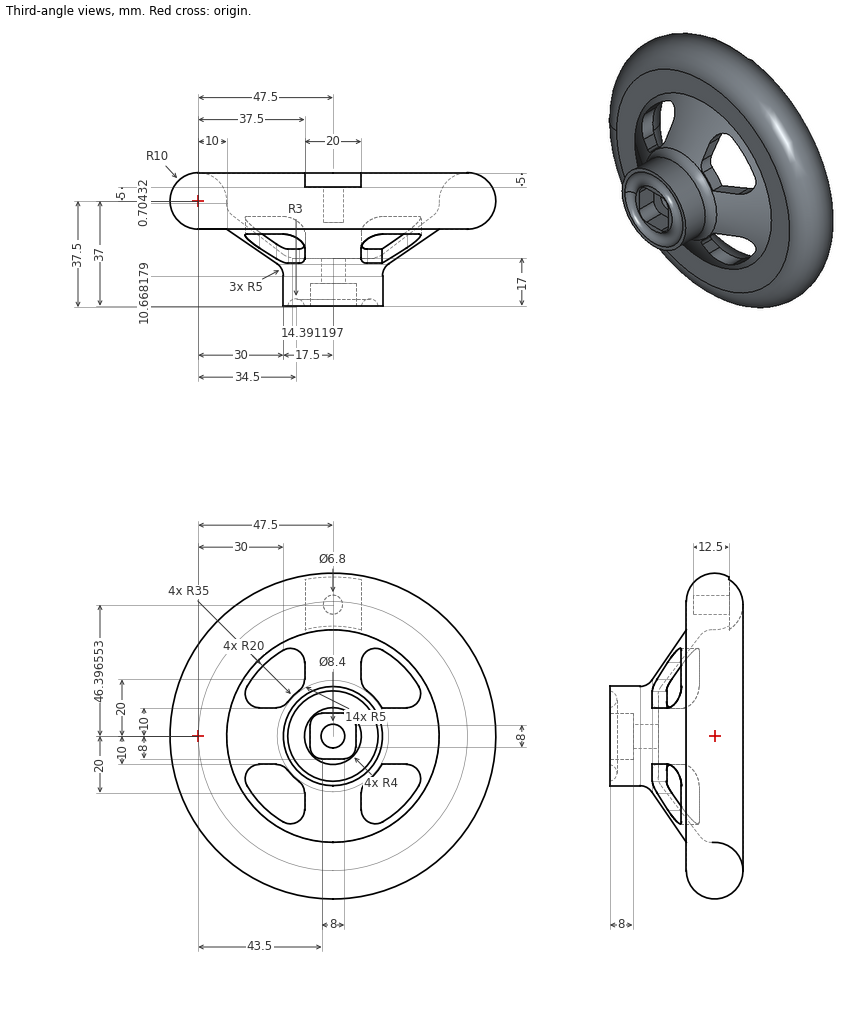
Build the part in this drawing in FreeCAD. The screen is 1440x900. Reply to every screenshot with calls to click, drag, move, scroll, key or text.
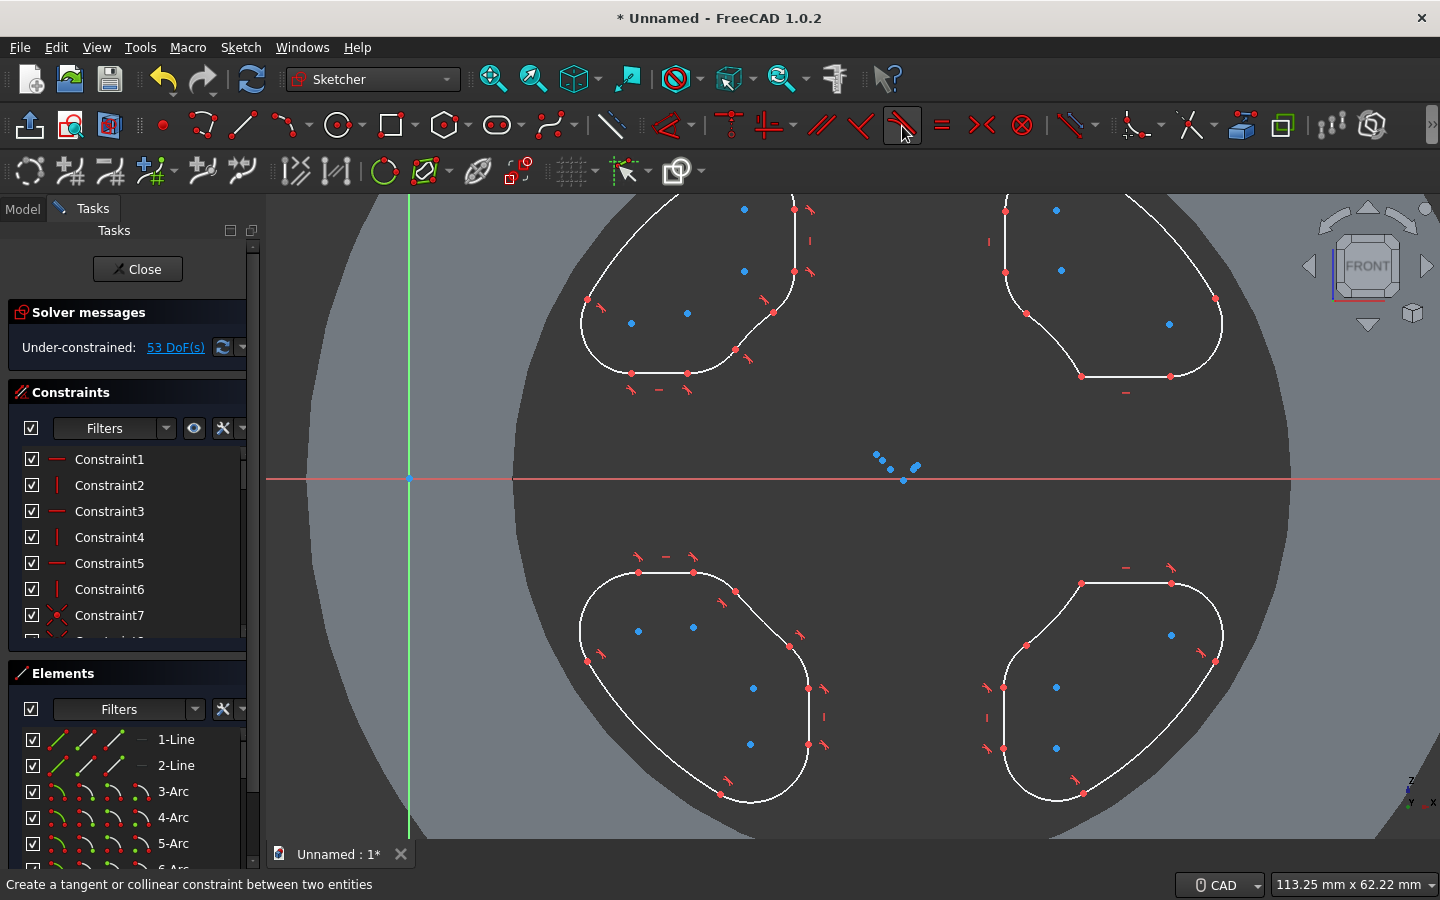
click(1015, 655)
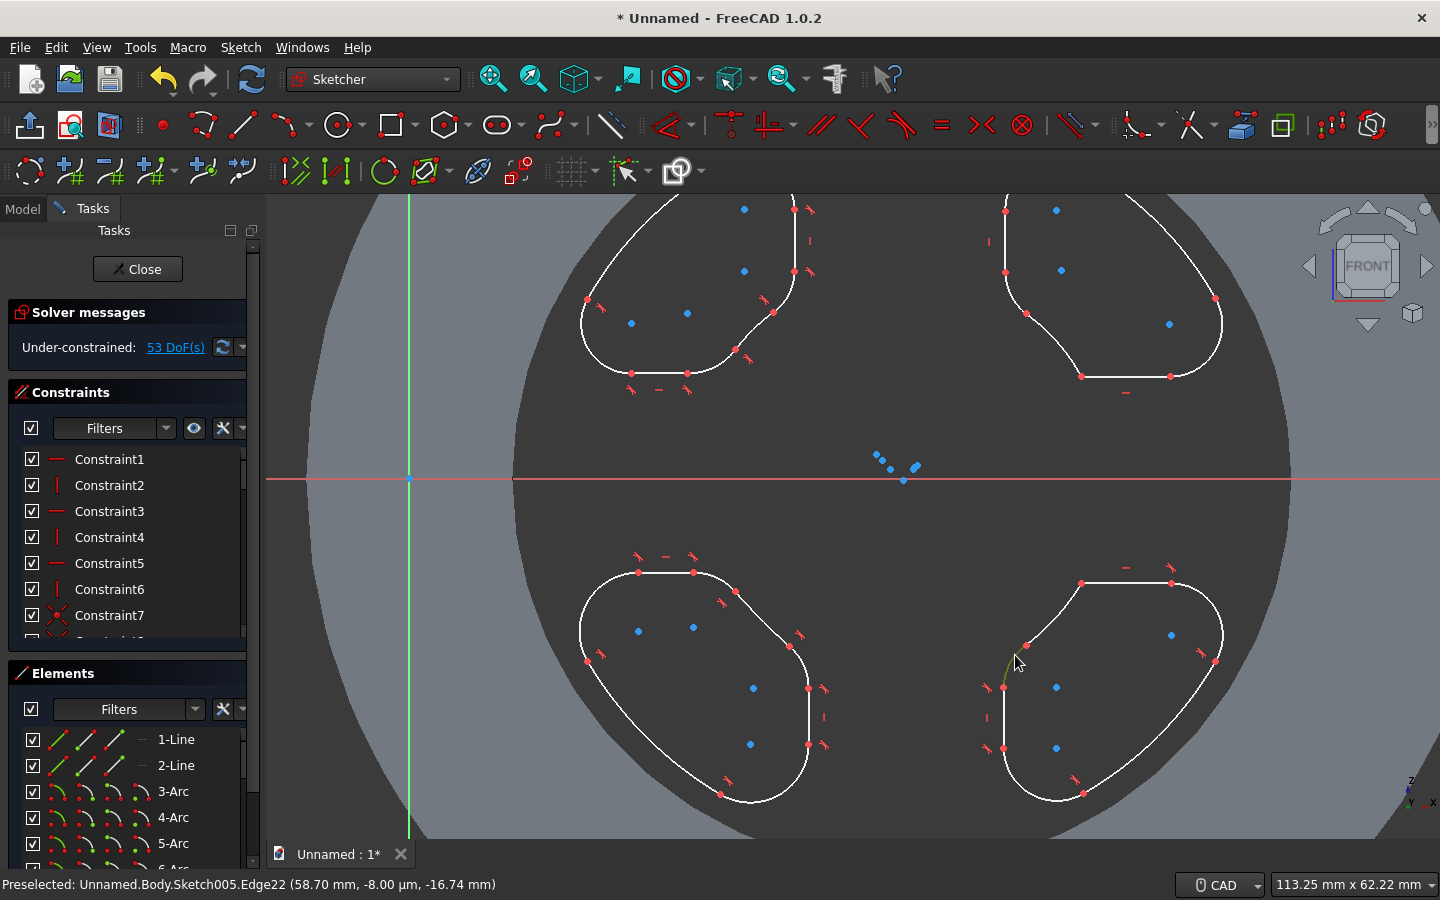
click(1045, 629)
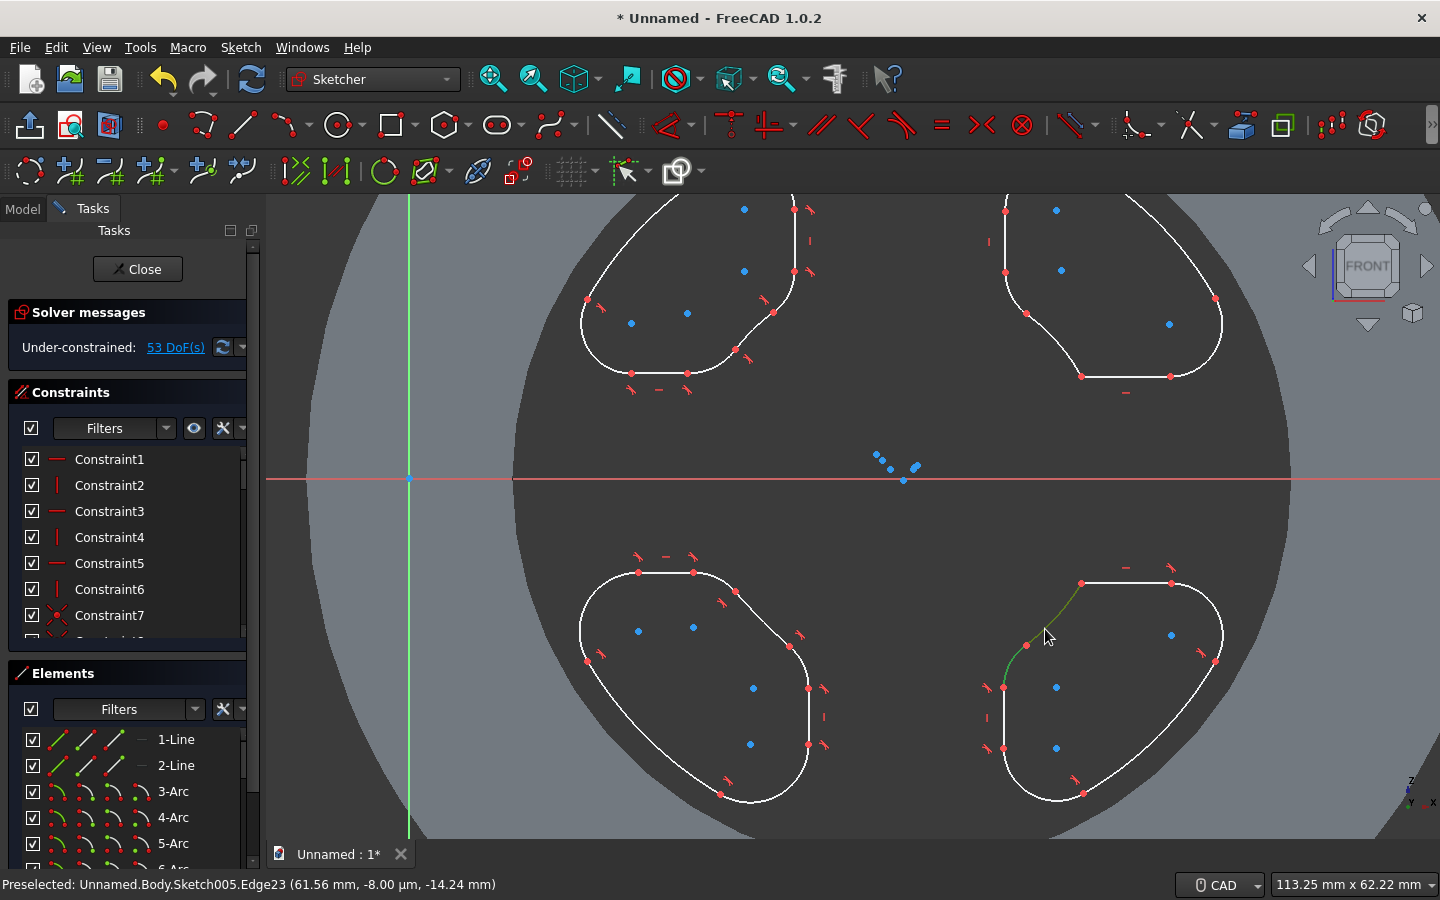
click(902, 126)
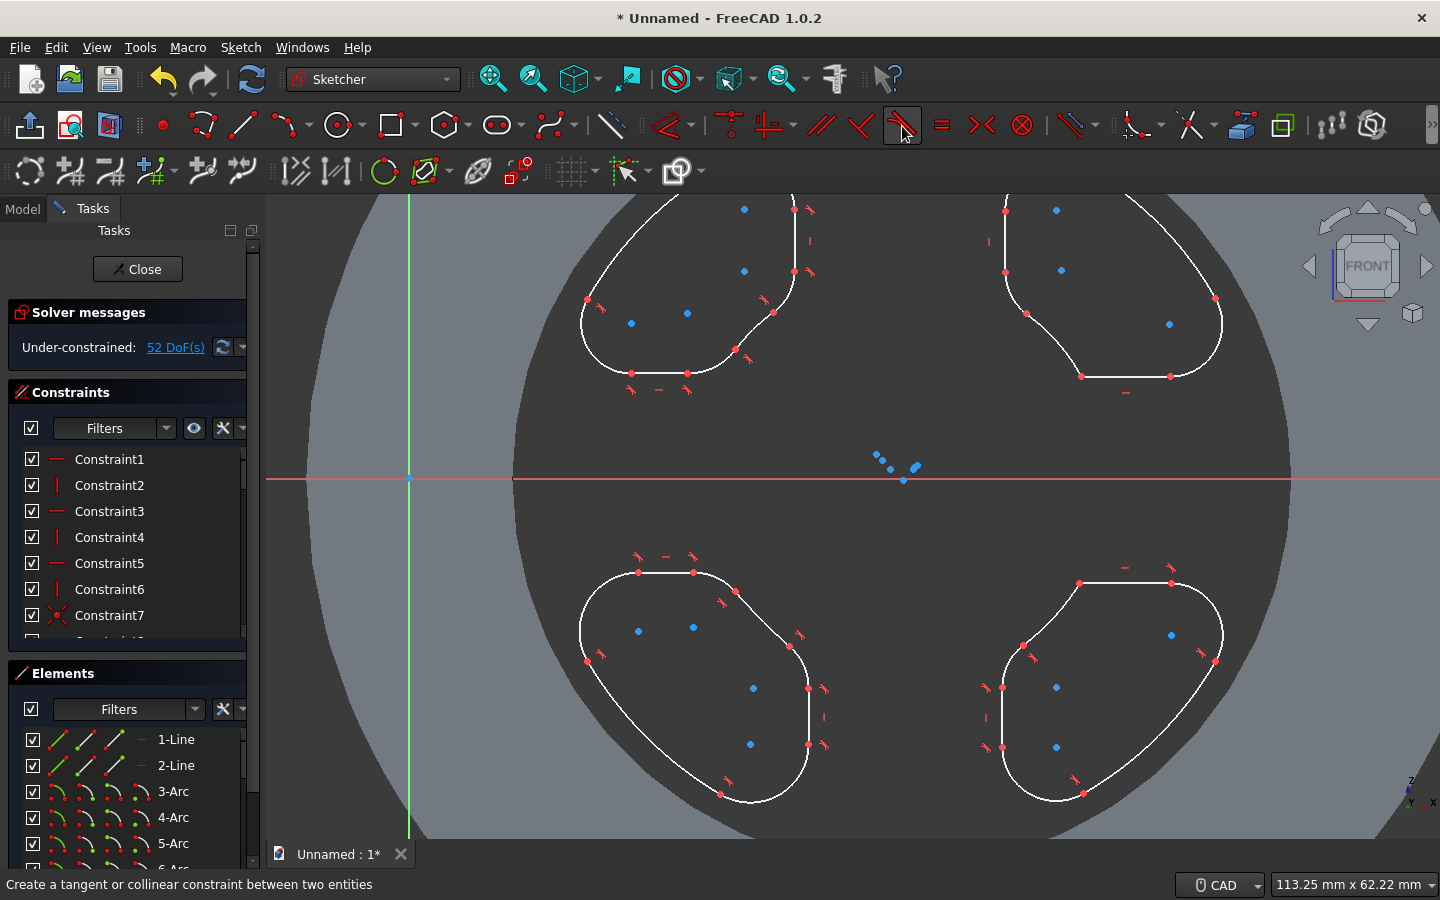
click(1144, 377)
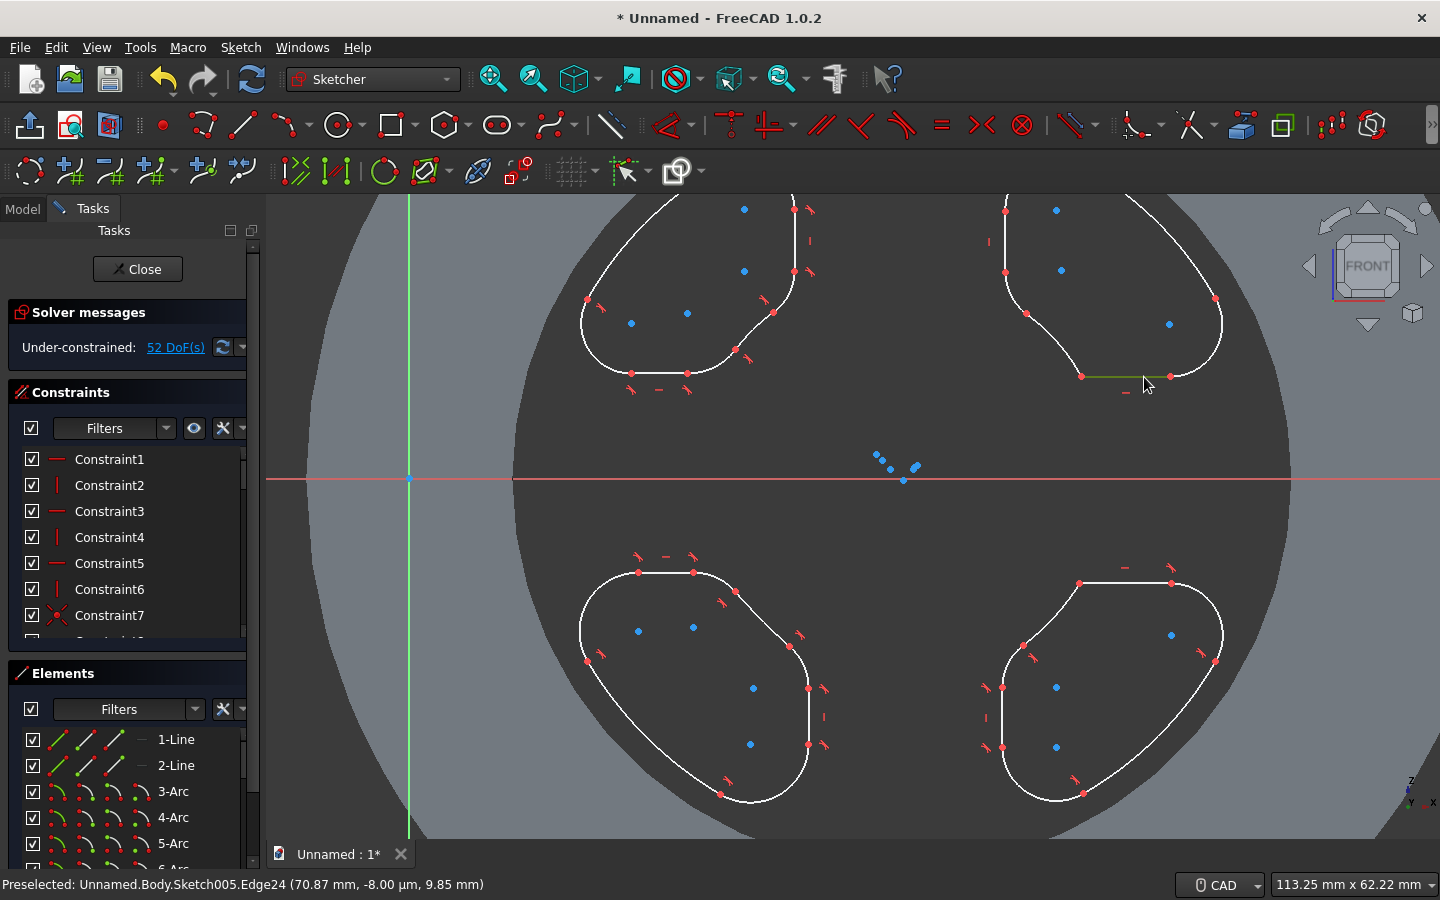
click(1201, 366)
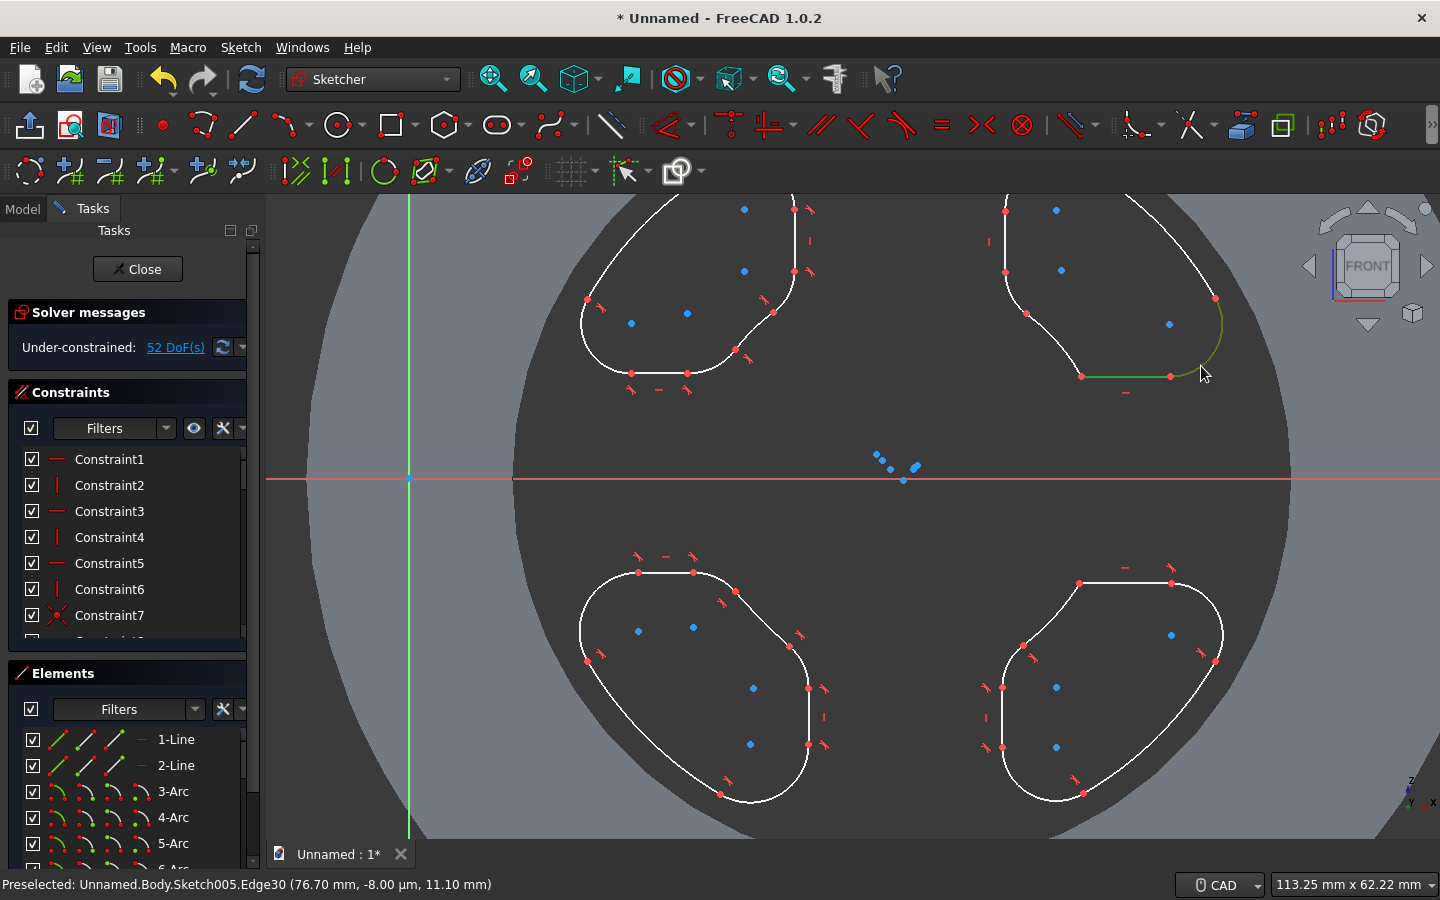
click(902, 126)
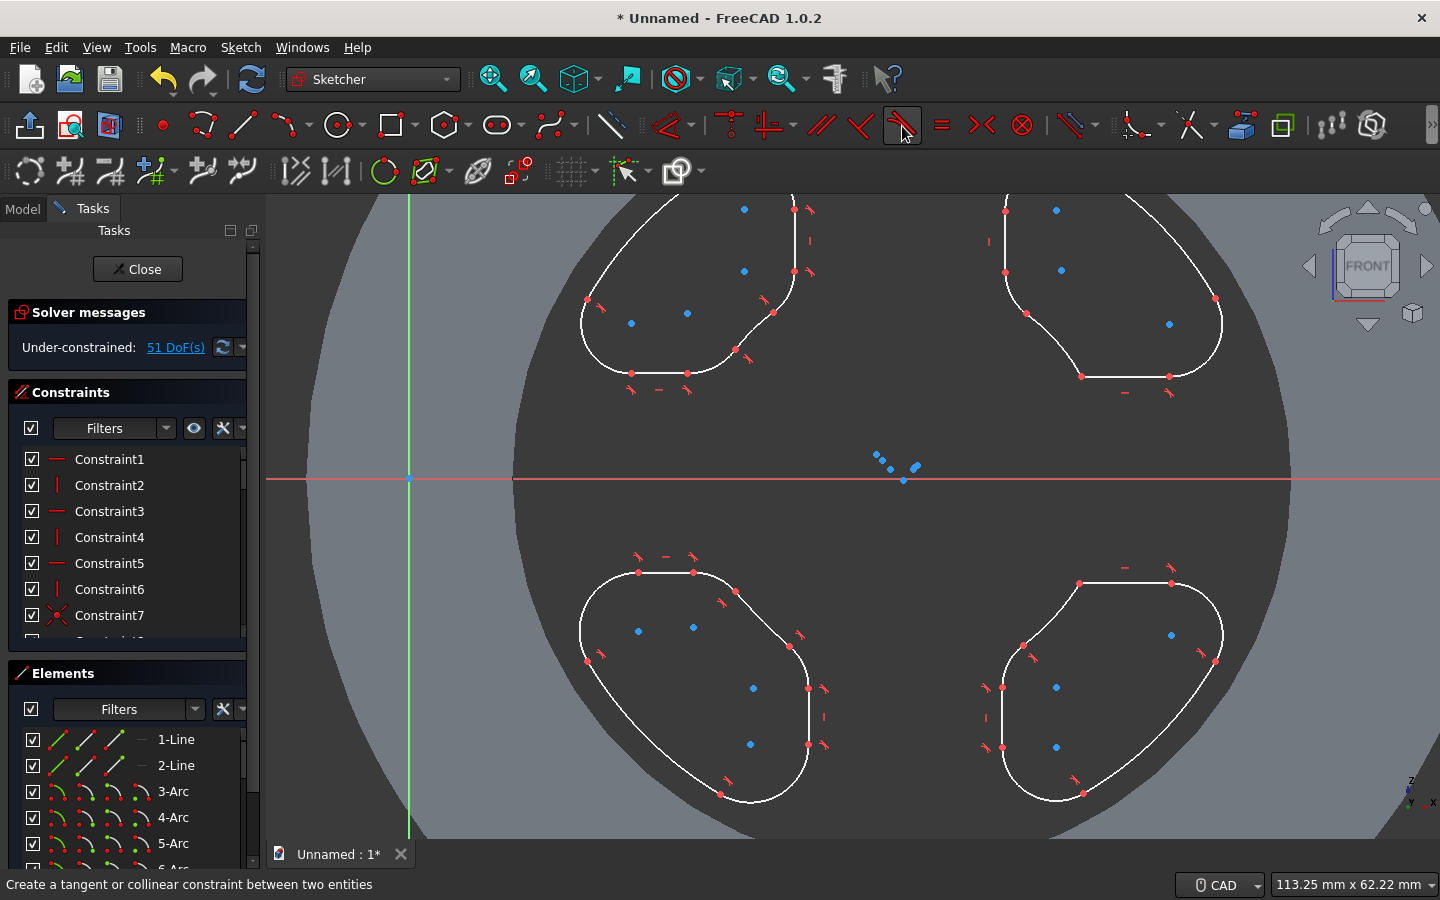
click(1005, 254)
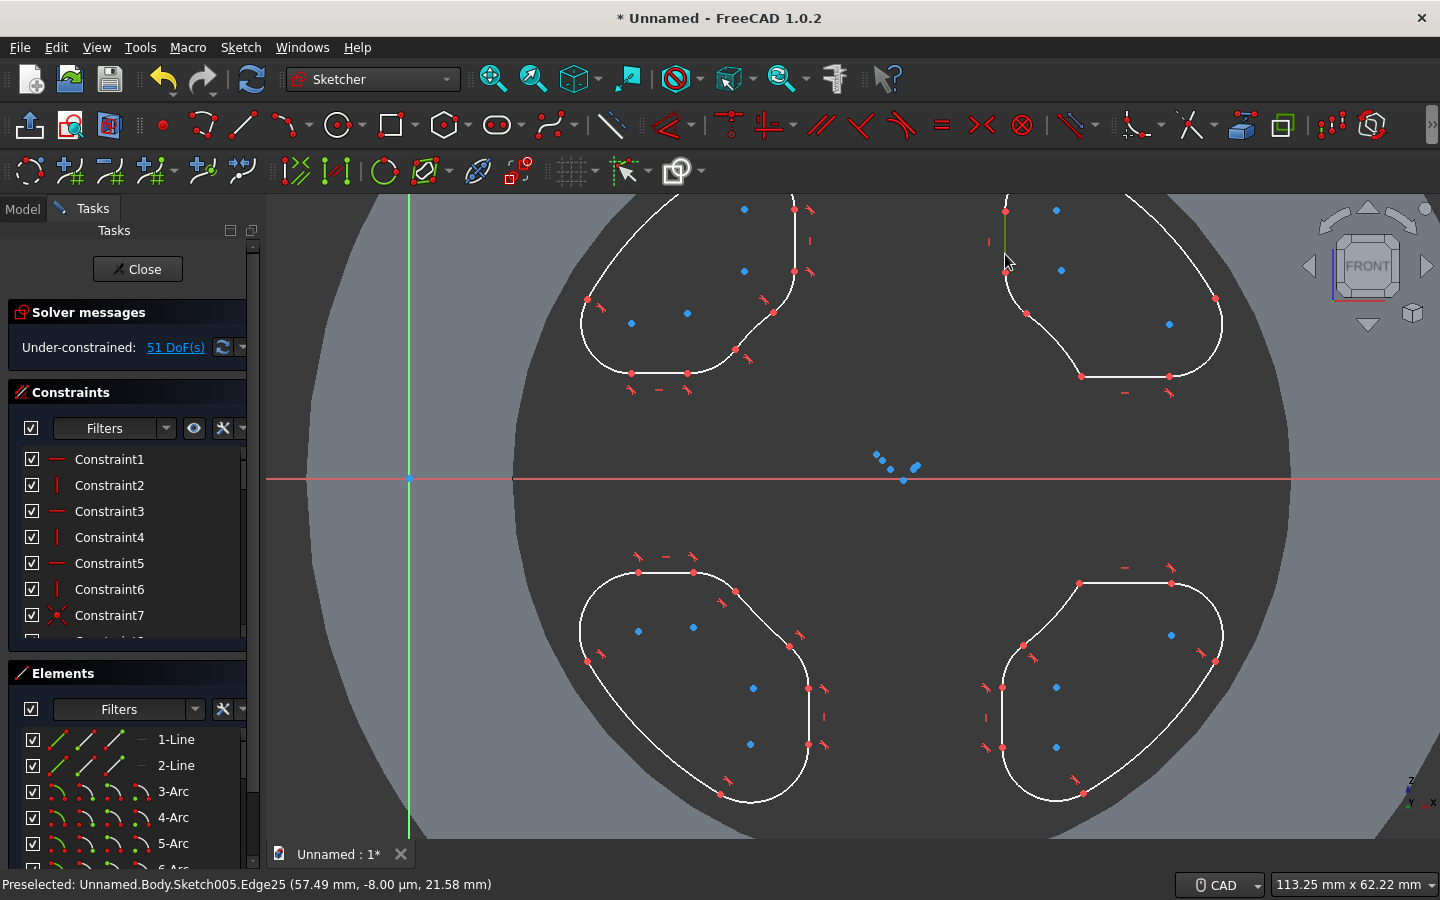
click(1008, 286)